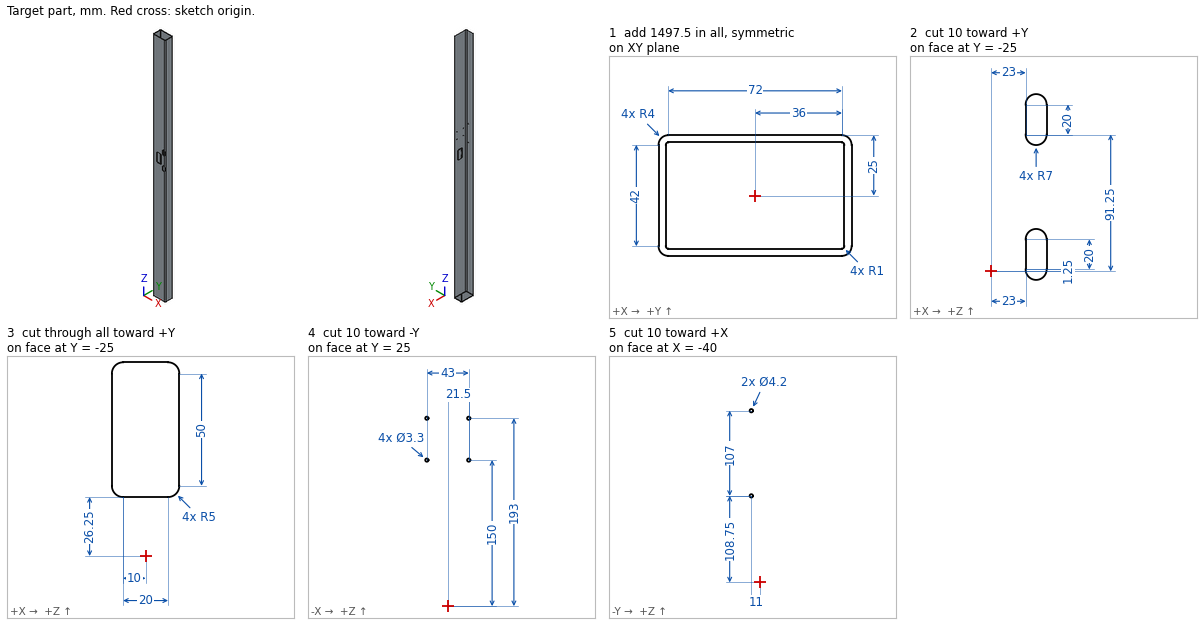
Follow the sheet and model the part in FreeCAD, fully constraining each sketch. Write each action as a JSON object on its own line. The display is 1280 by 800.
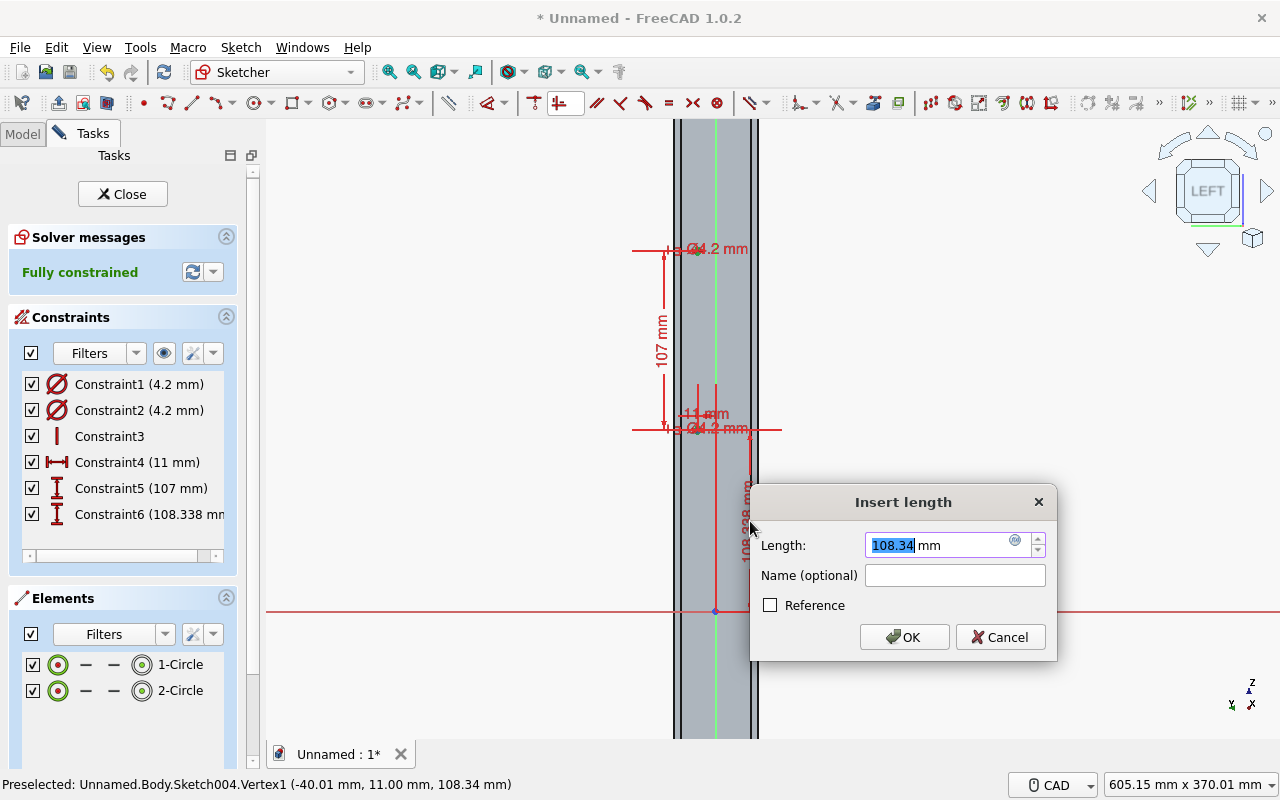
{"action": "type", "text": "108.75"}
{"action": "key", "text": "Return"}
{"action": "key", "text": "Escape"}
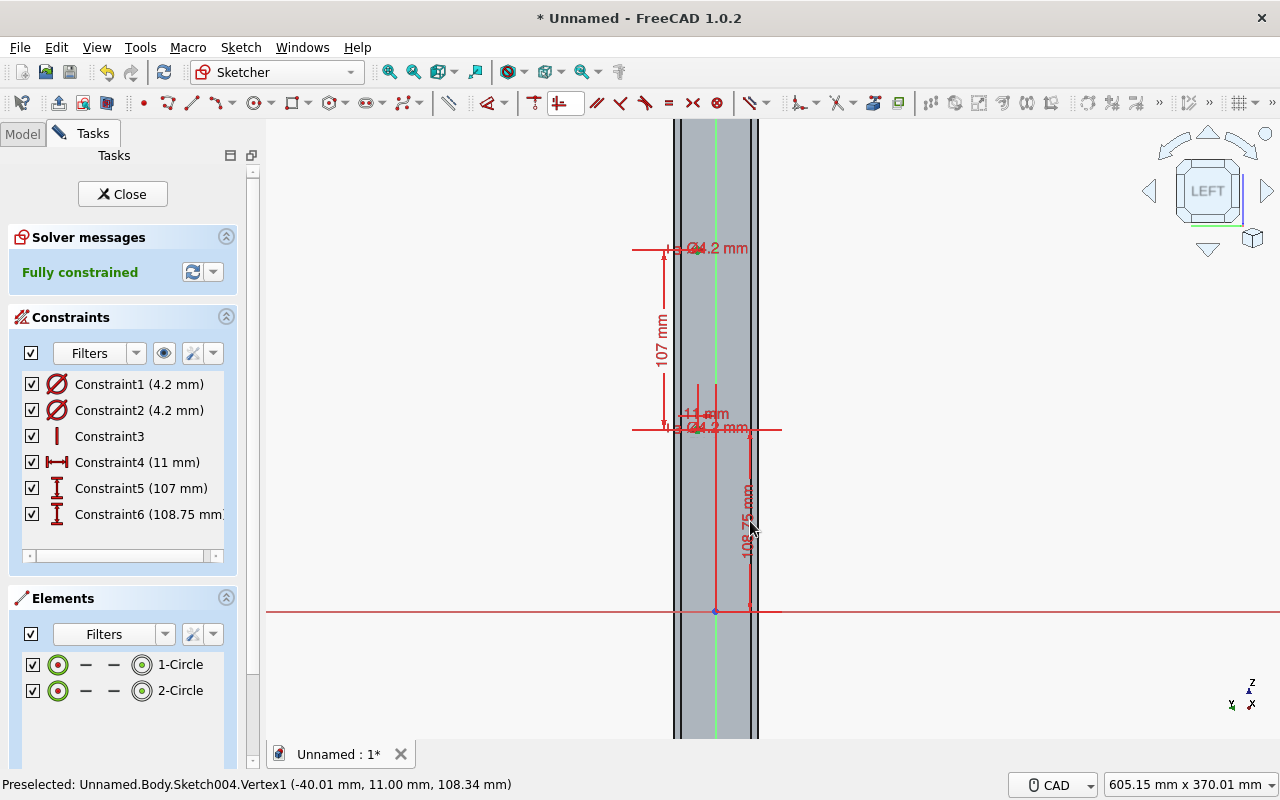
{"action": "left_click", "coordinate": [123, 194]}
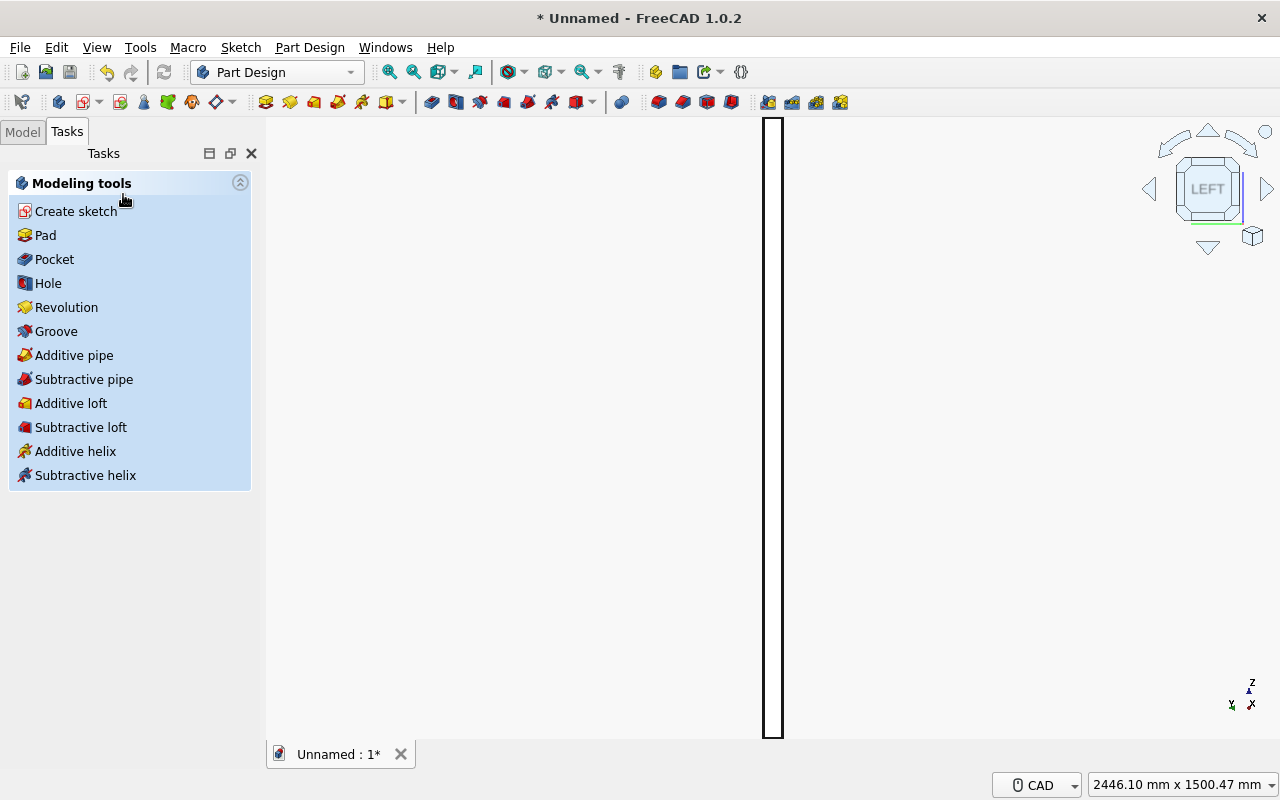
{"action": "left_click", "coordinate": [432, 102]}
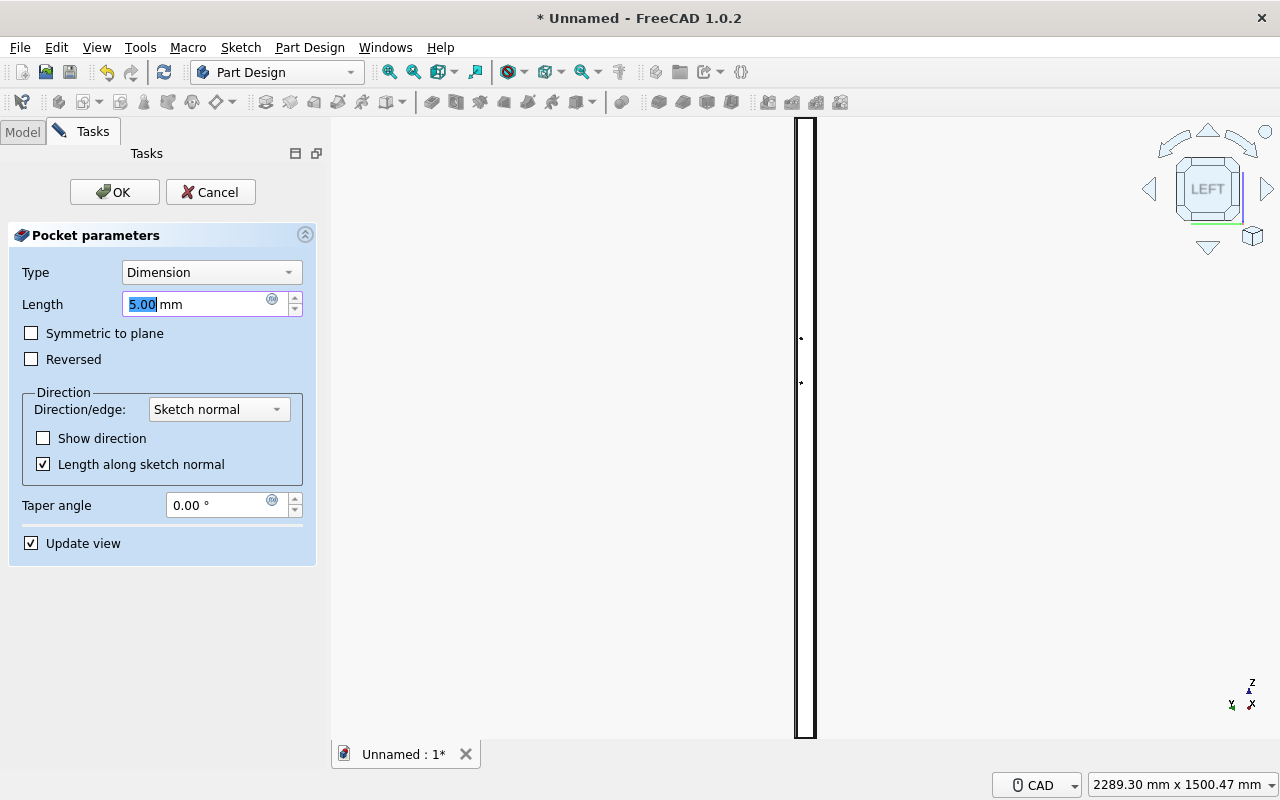
{"action": "type", "text": "10"}
{"action": "key", "text": "Tab"}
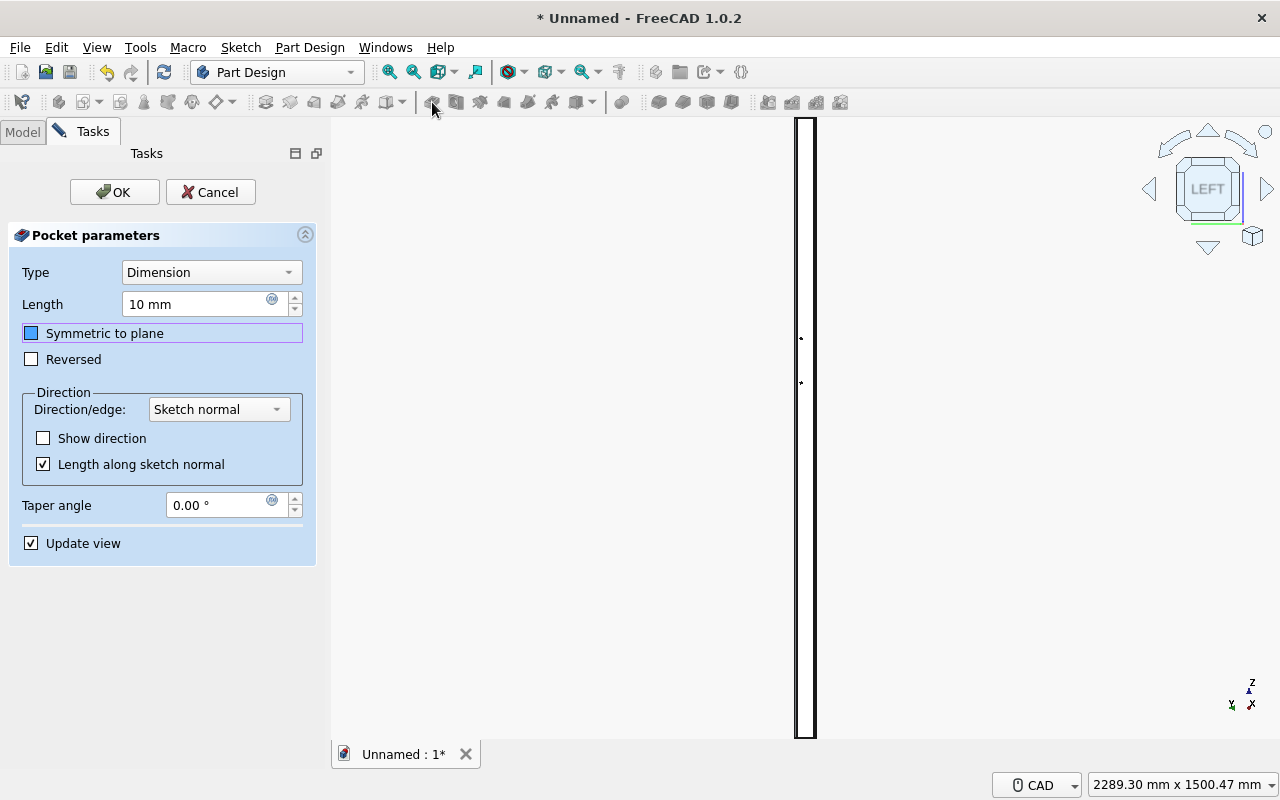
{"action": "left_click", "coordinate": [115, 192]}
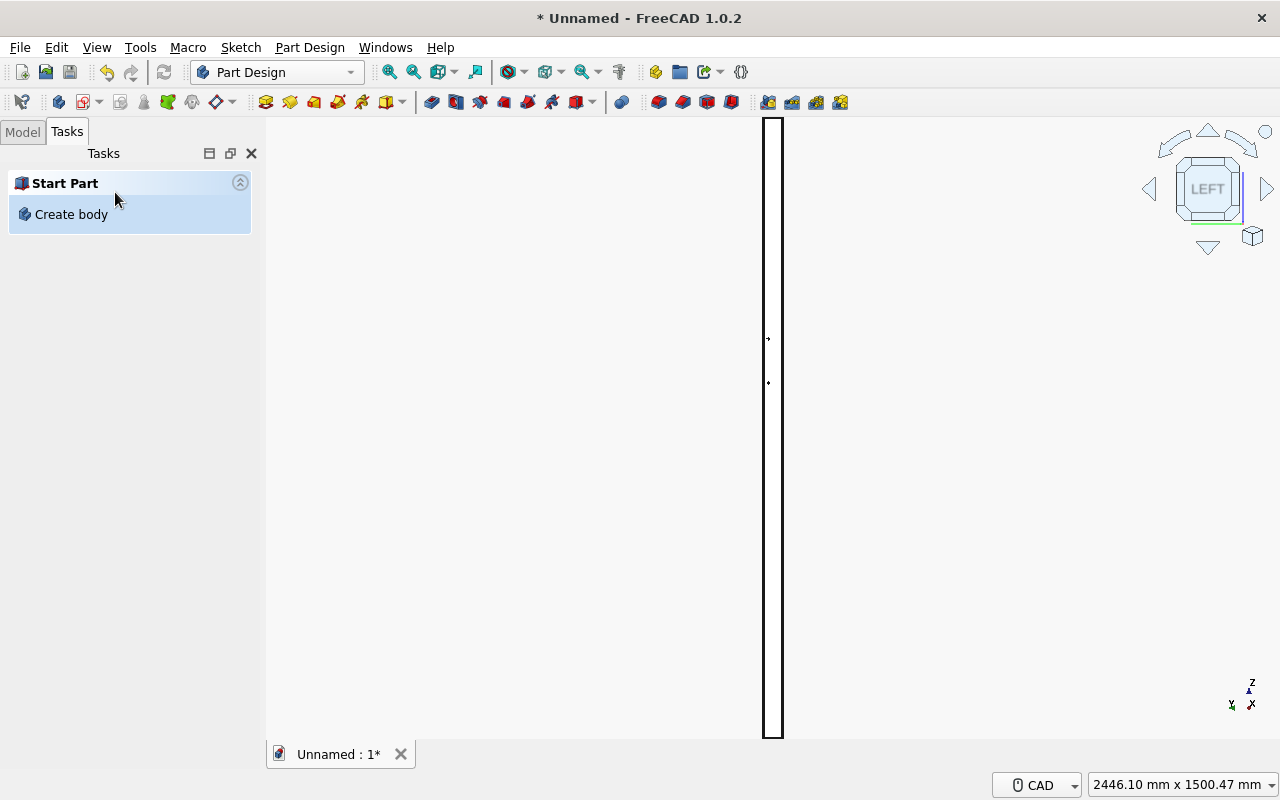
{"action": "key", "text": "0"}